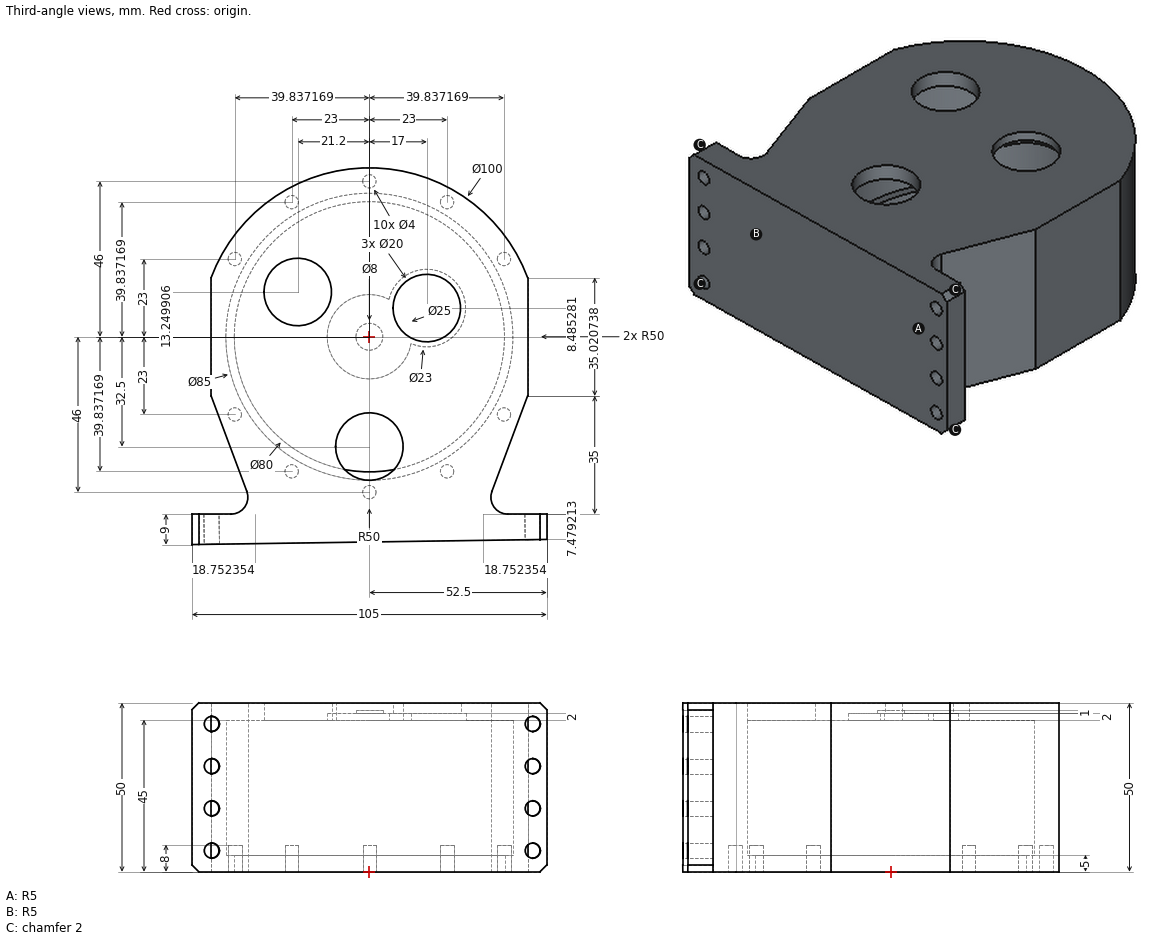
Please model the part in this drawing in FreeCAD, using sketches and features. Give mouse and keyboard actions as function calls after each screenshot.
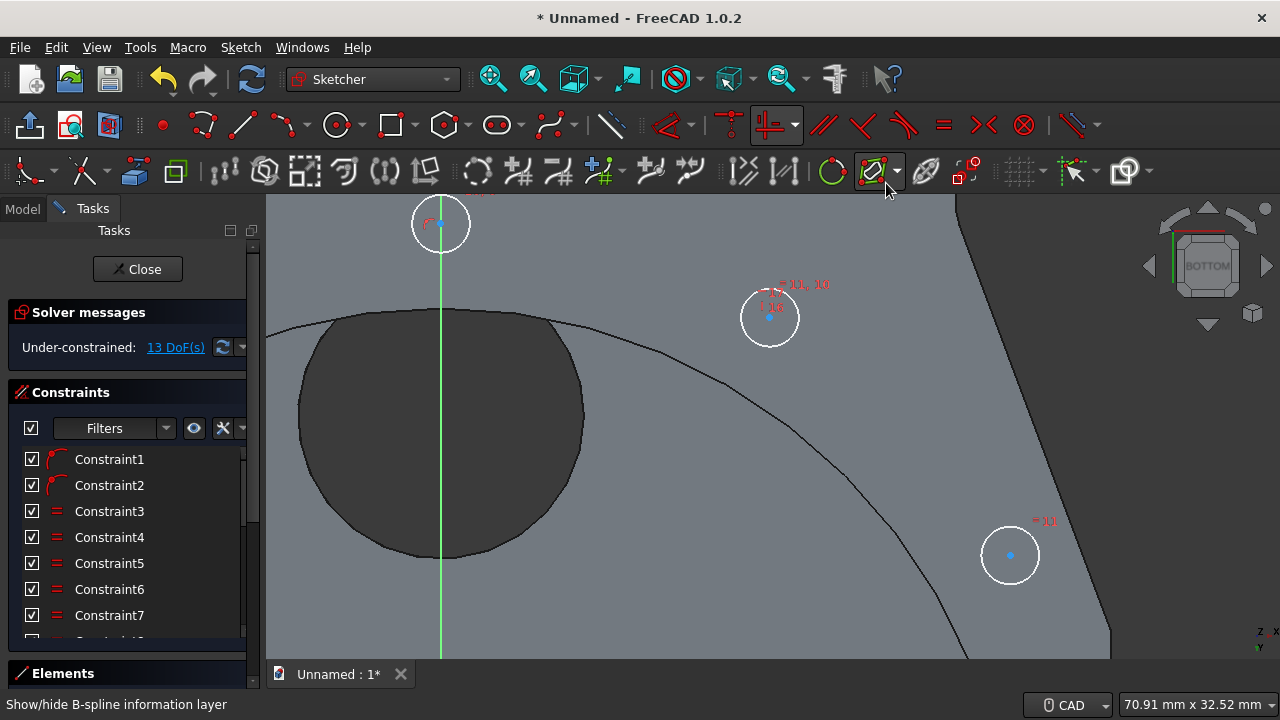
scroll(771, 312, down, 8)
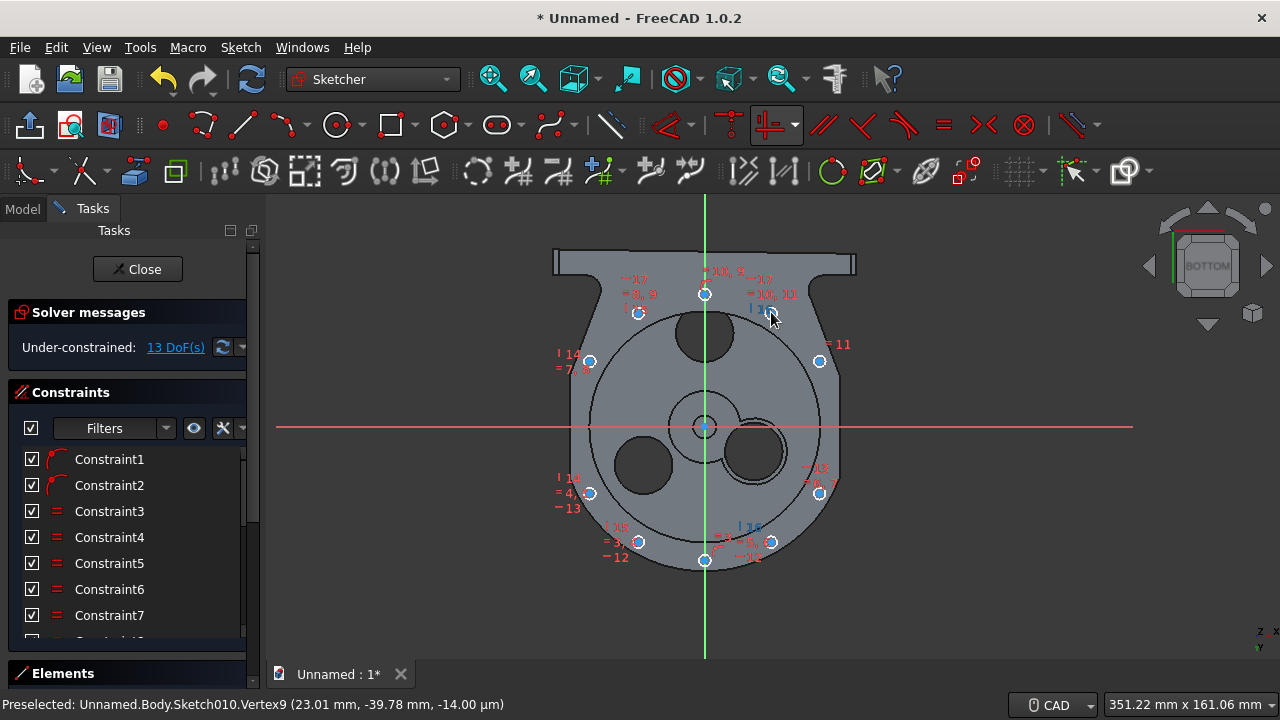
click(820, 494)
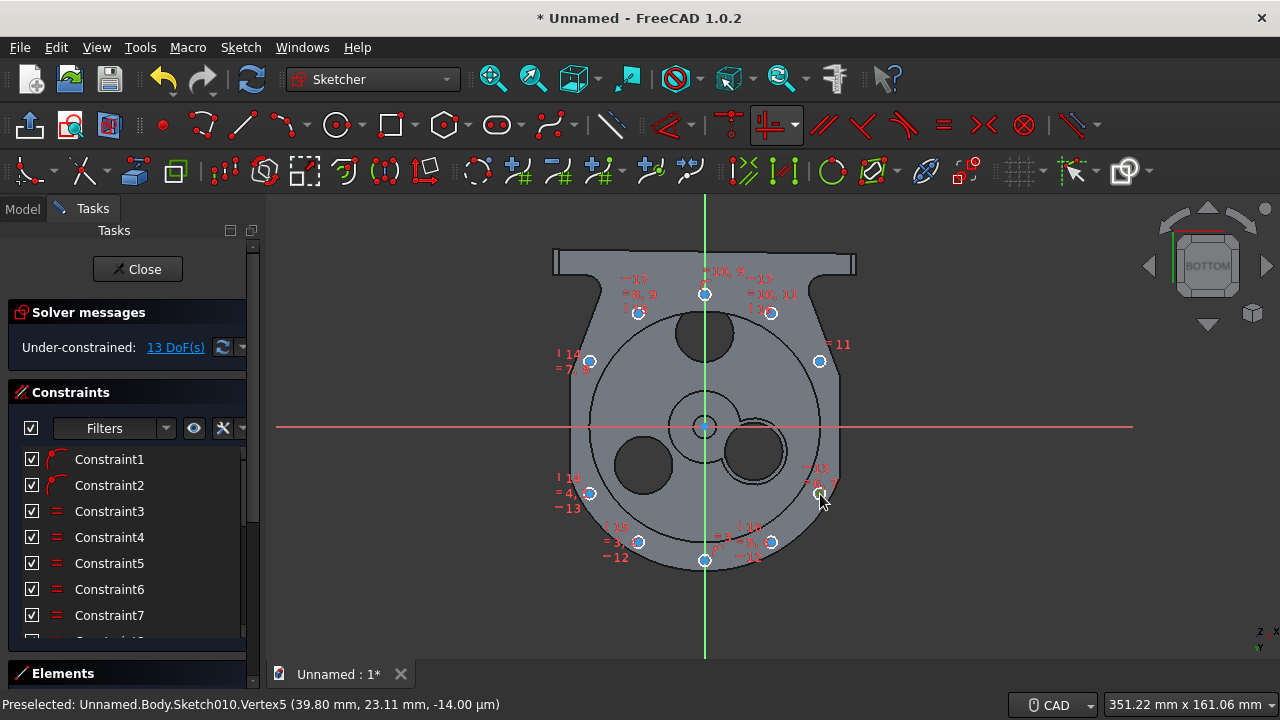
click(820, 361)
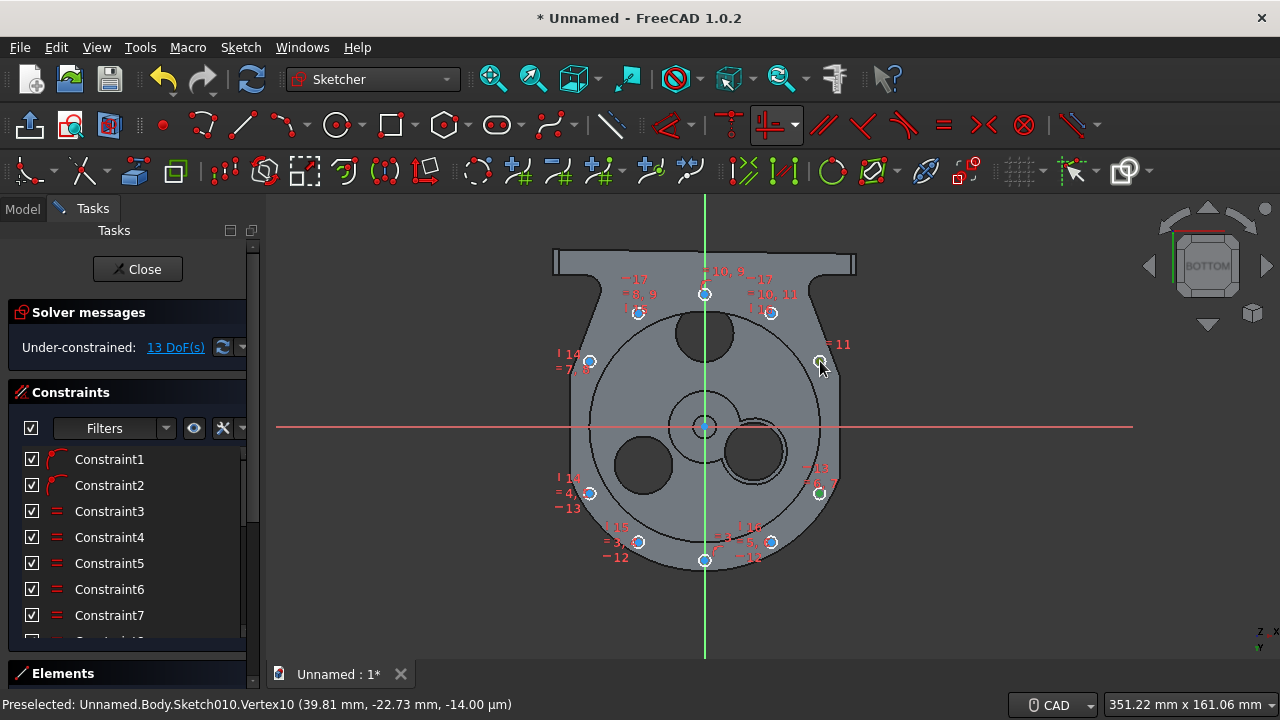
key(v)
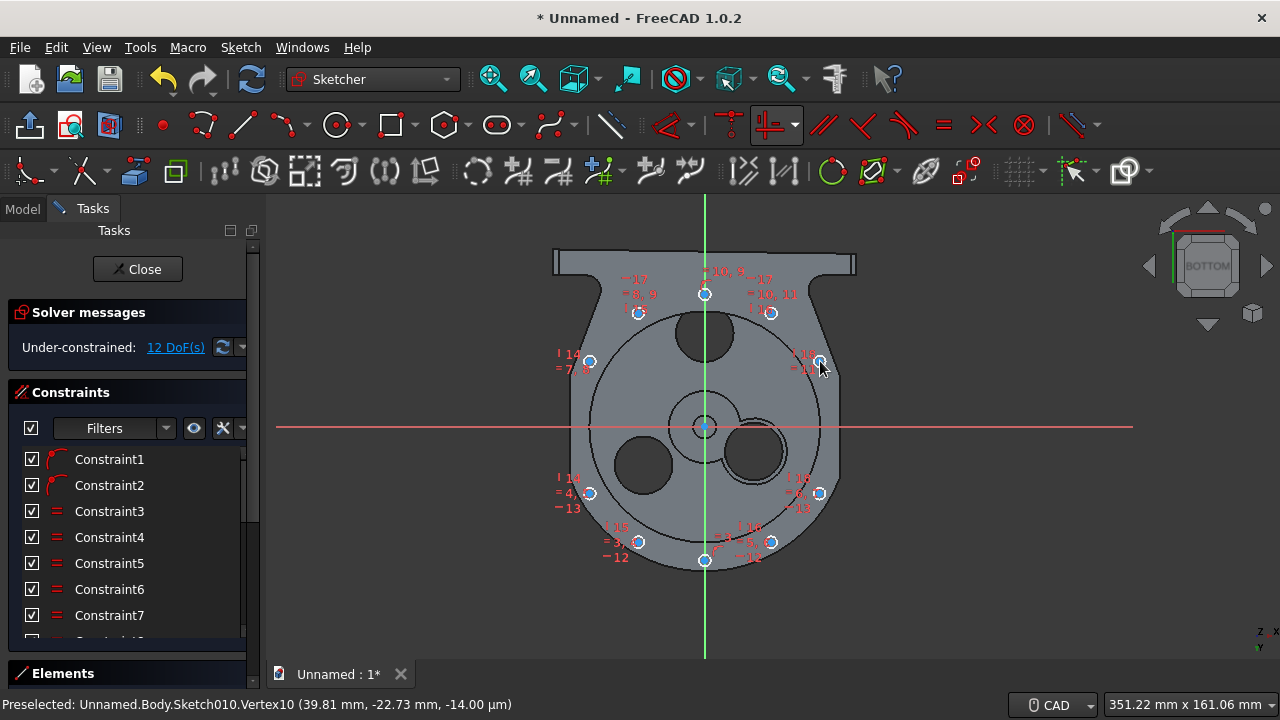
click(590, 361)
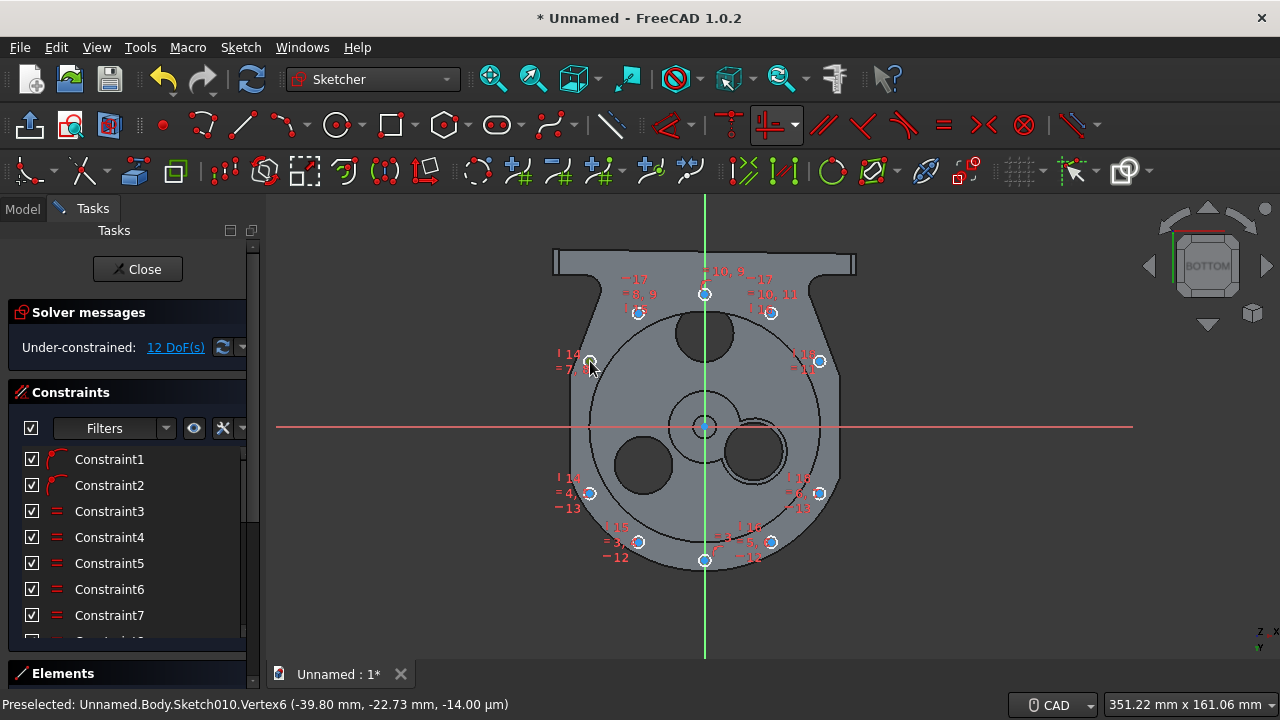
click(820, 361)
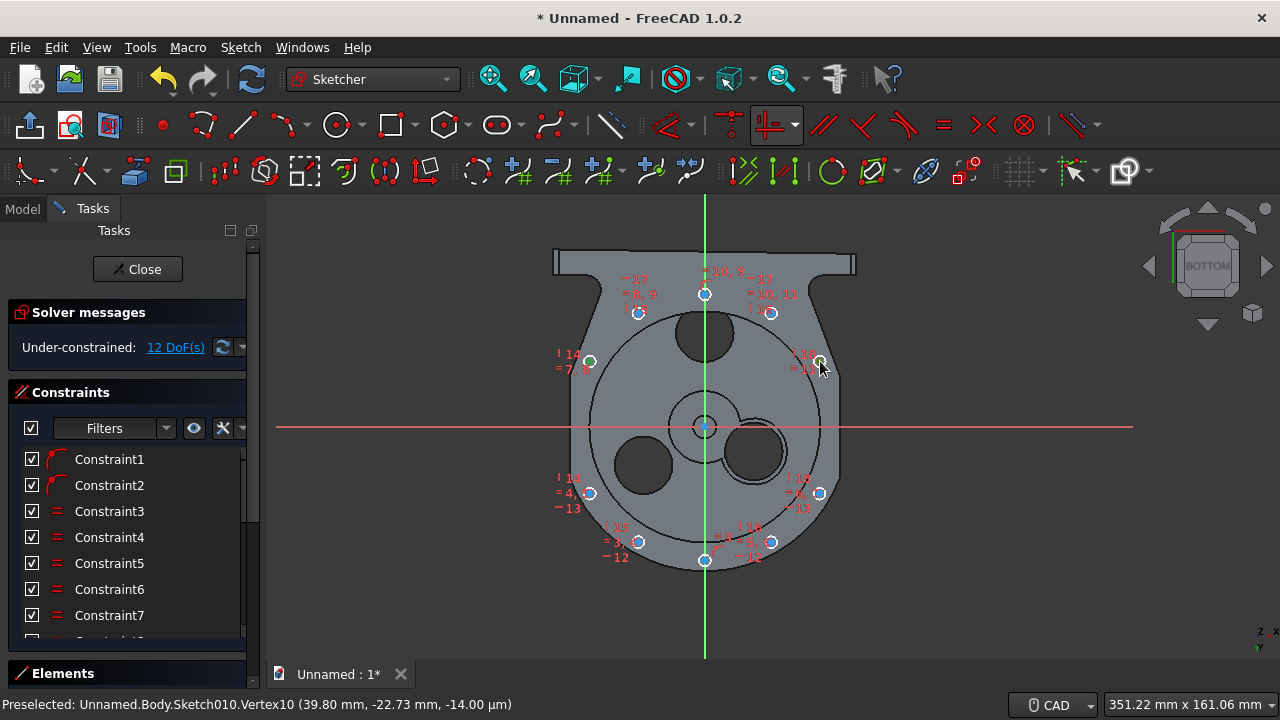
click(798, 126)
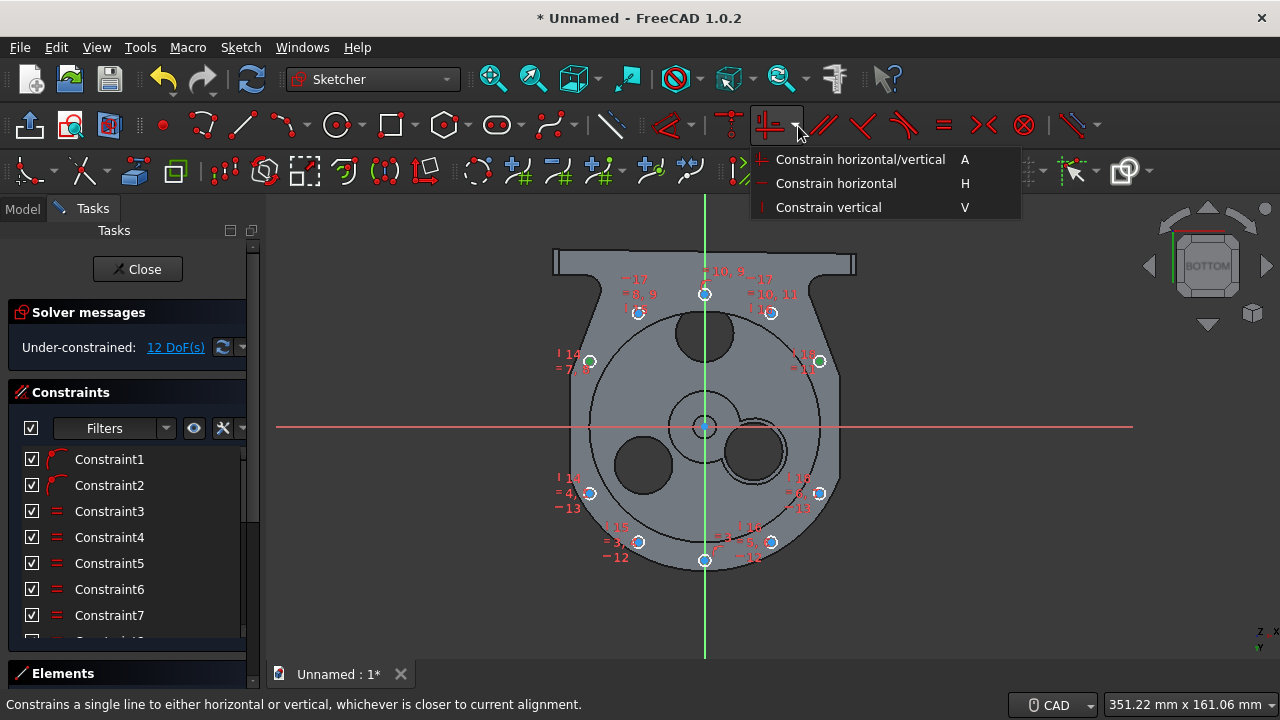
click(886, 183)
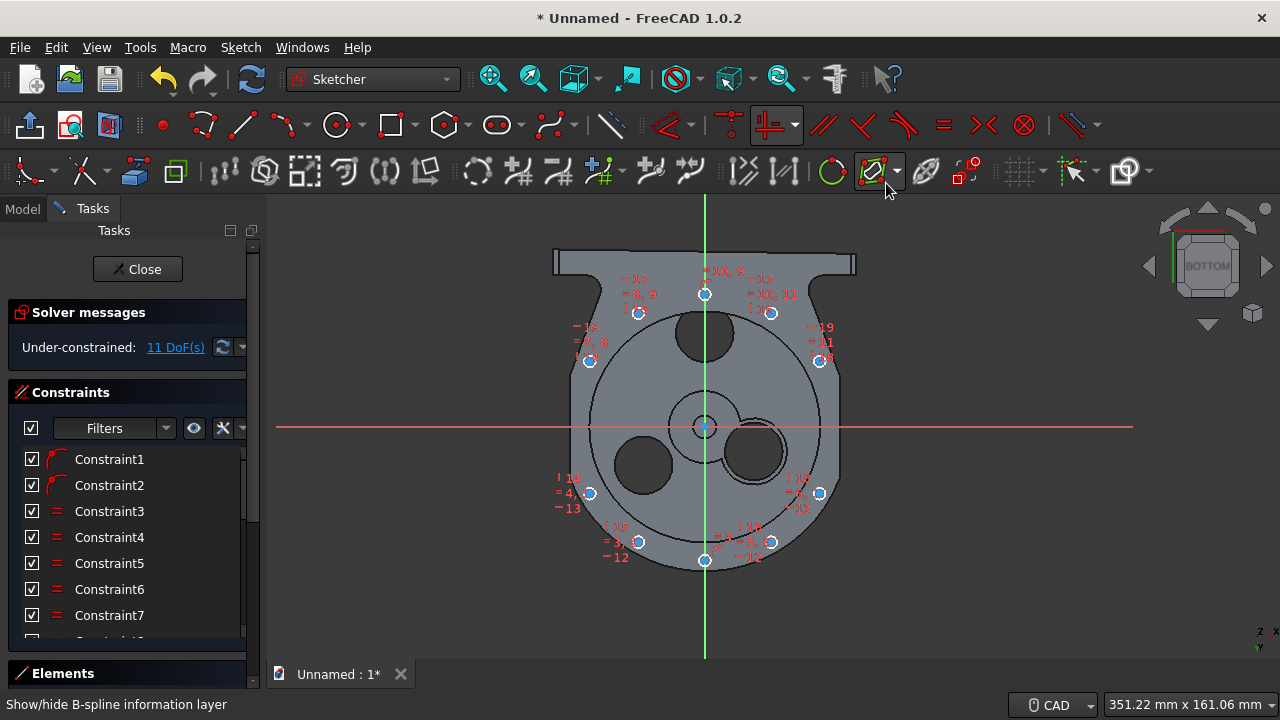
click(666, 126)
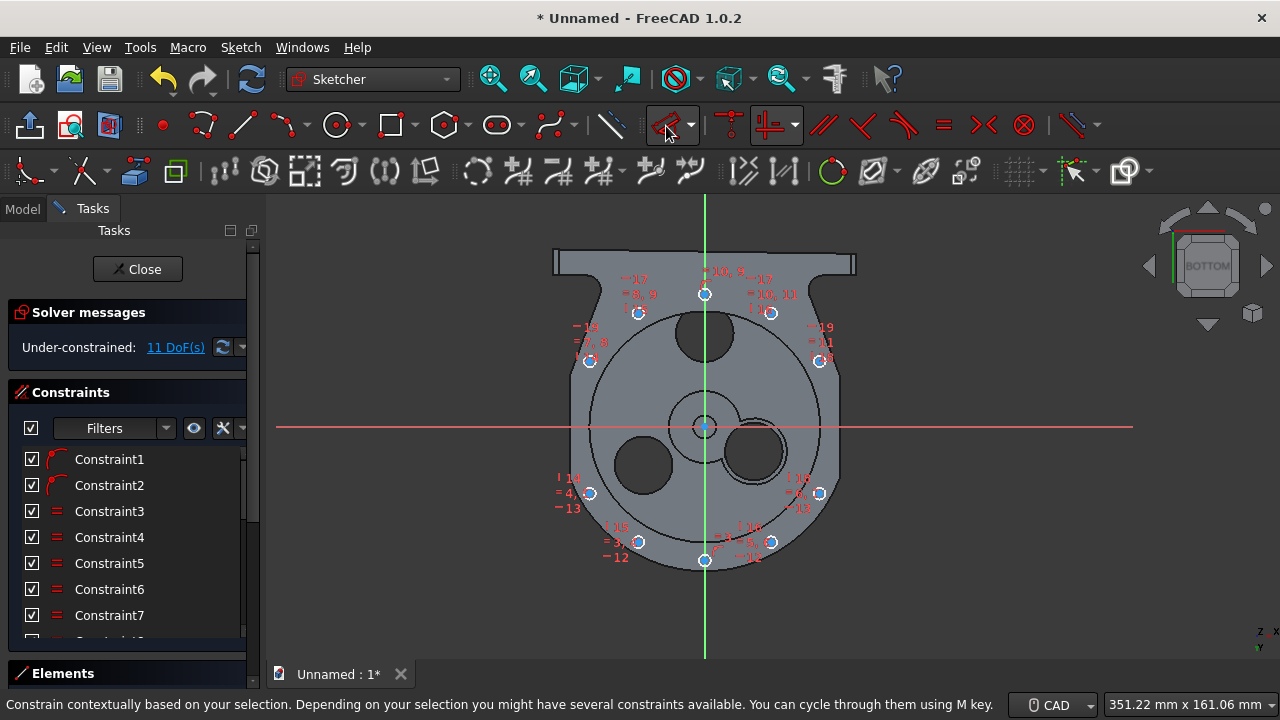
scroll(705, 555, up, 7)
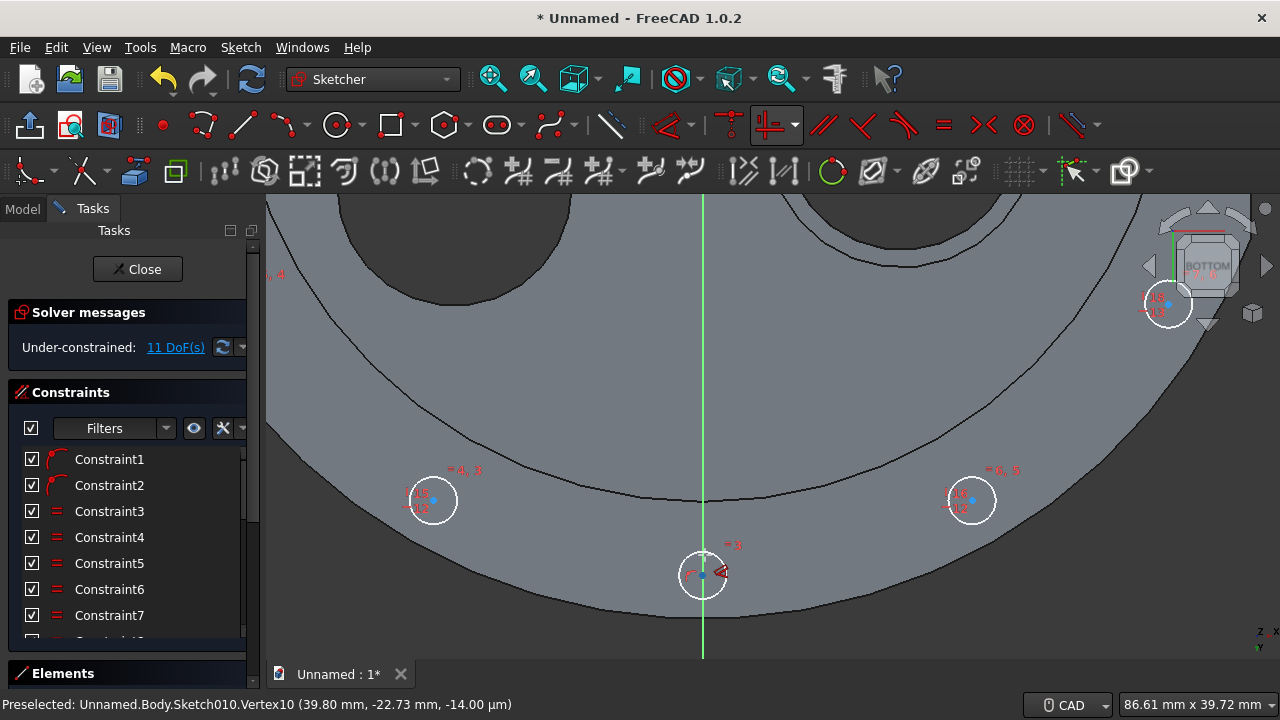
click(703, 552)
click(730, 527)